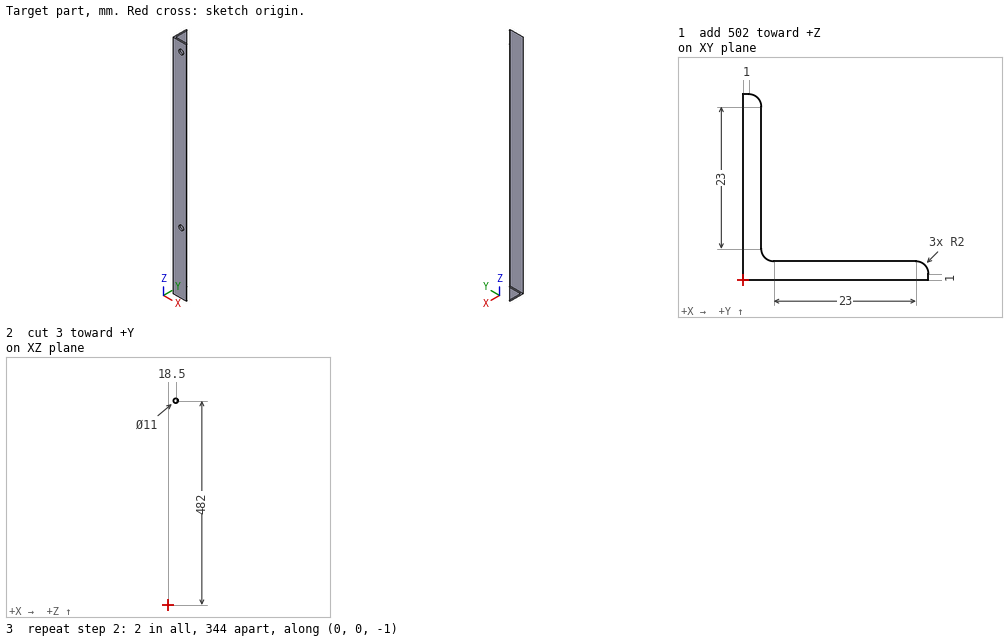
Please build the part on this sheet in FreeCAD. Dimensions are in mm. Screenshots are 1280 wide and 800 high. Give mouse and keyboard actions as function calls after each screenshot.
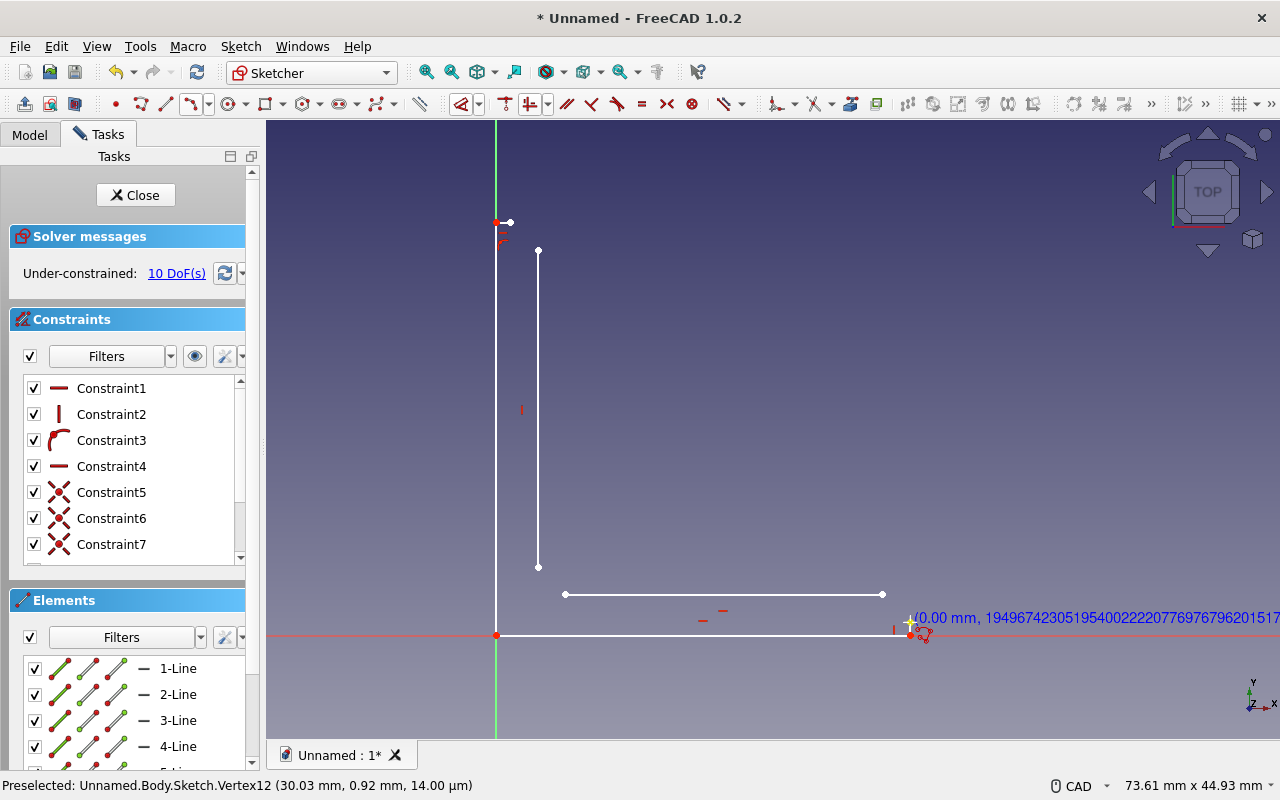
key(g)
key(3)
key(a)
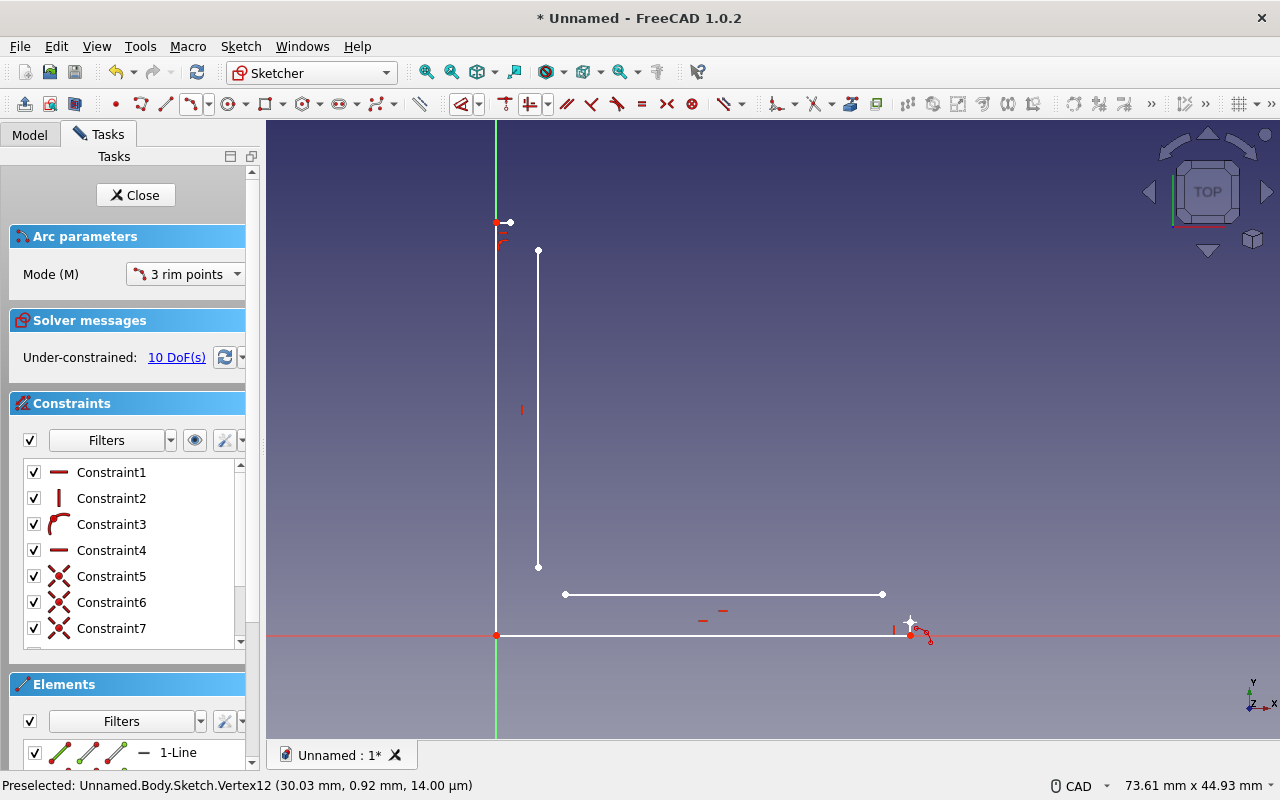
click(565, 595)
click(538, 568)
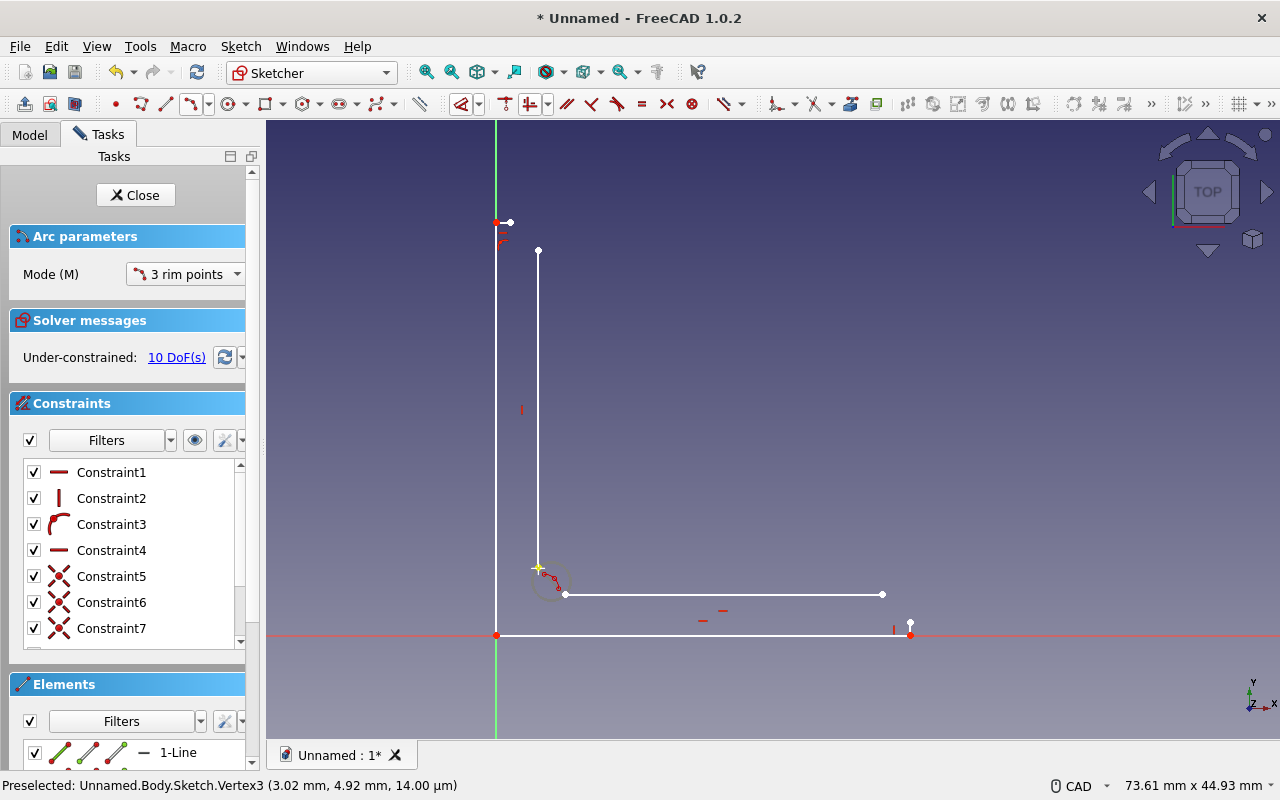
scroll(546, 586, up, 4)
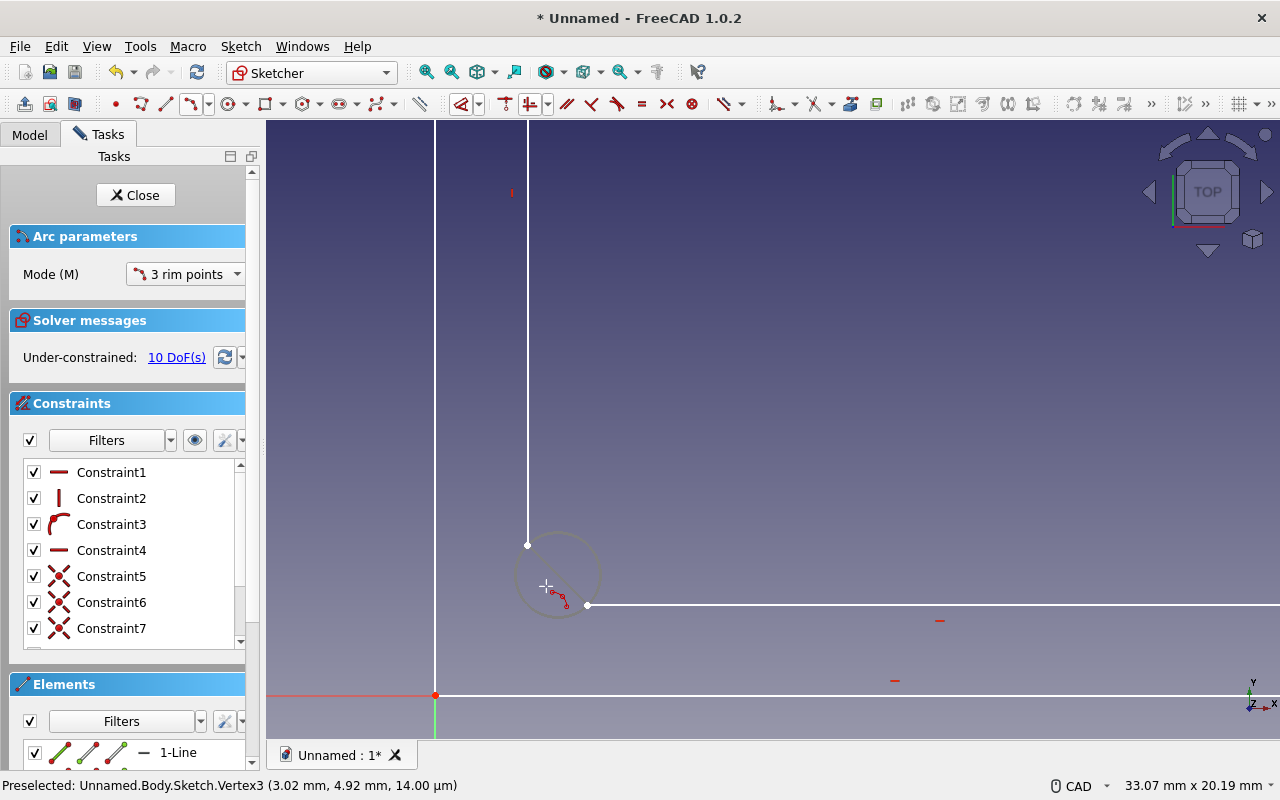
click(545, 586)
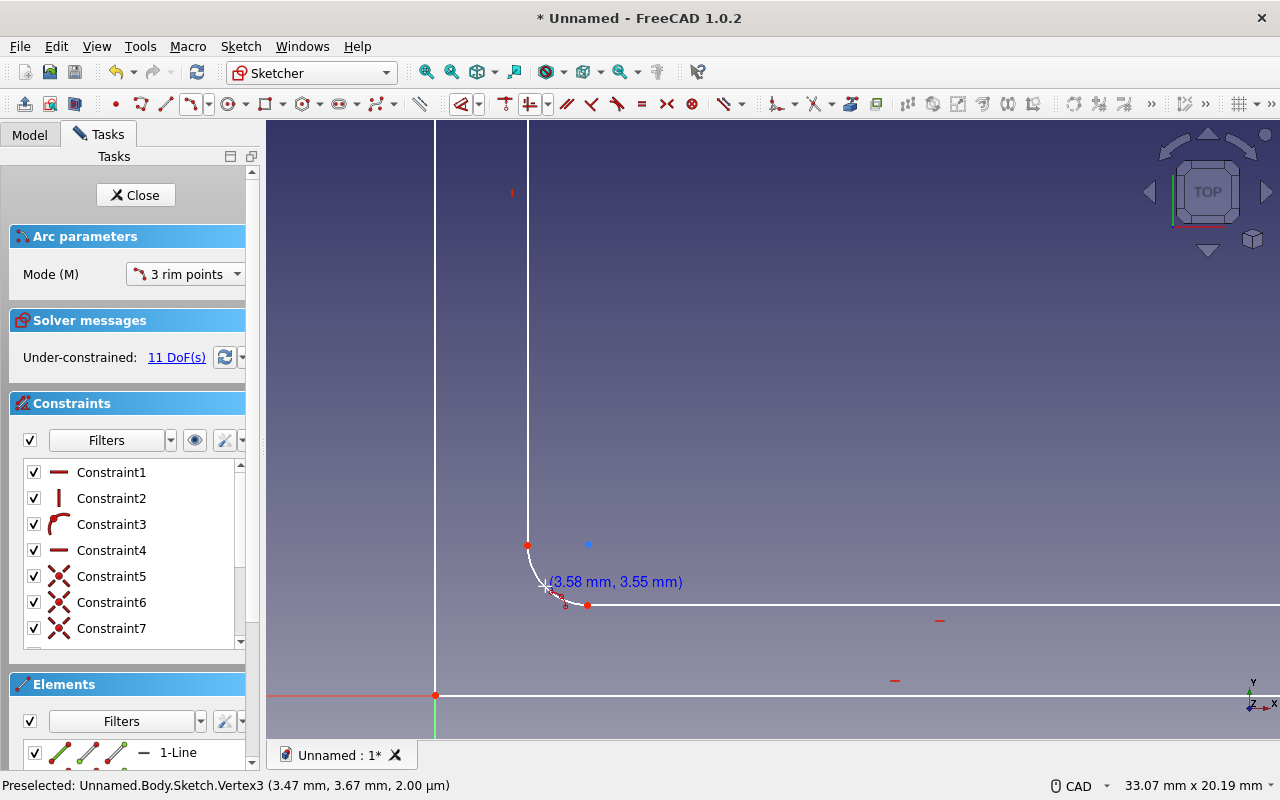
scroll(549, 588, down, 4)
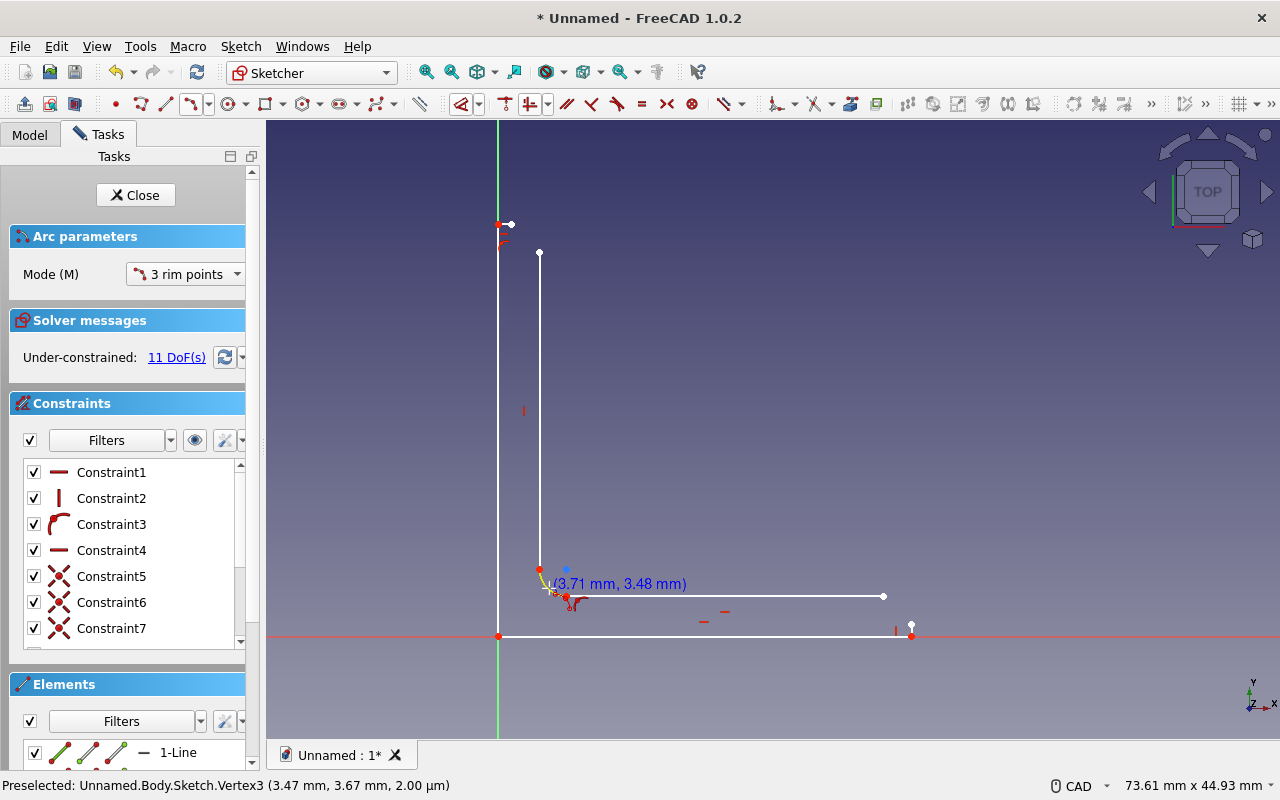
click(540, 252)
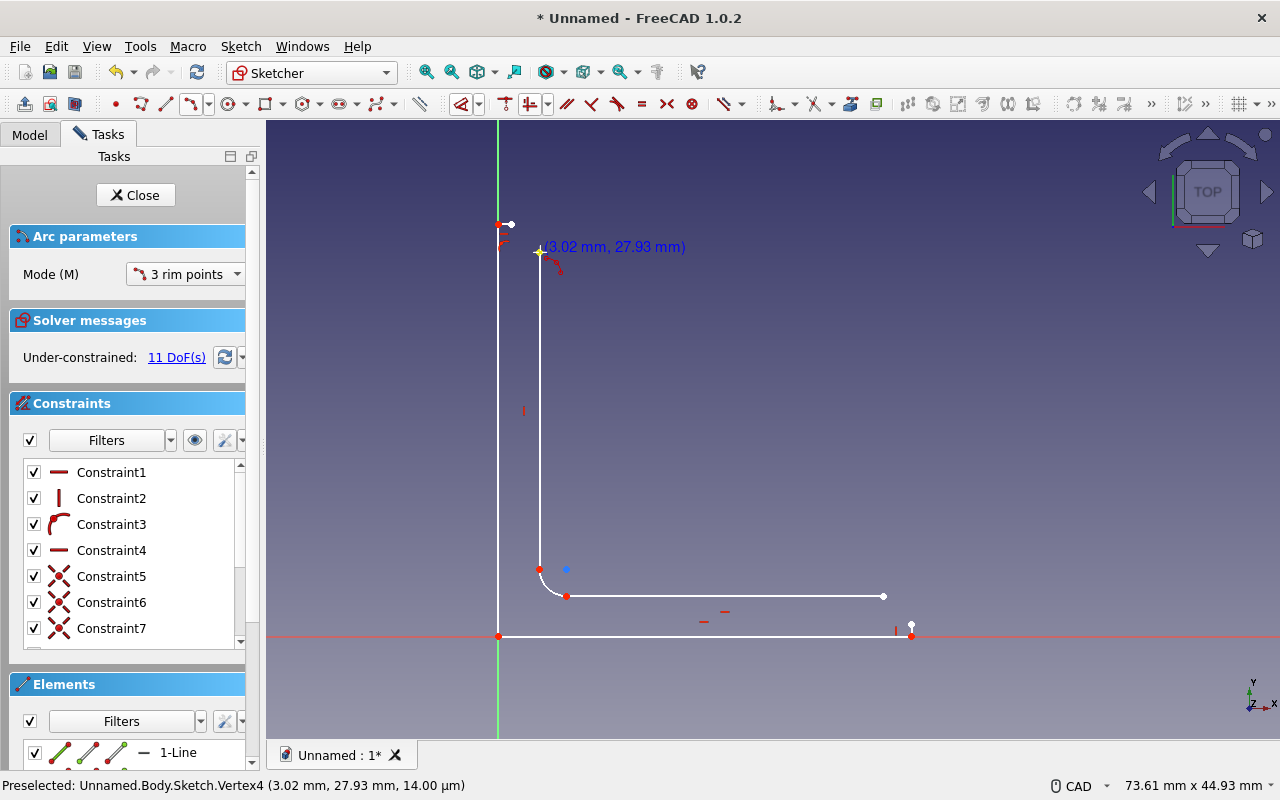
scroll(512, 224, up, 5)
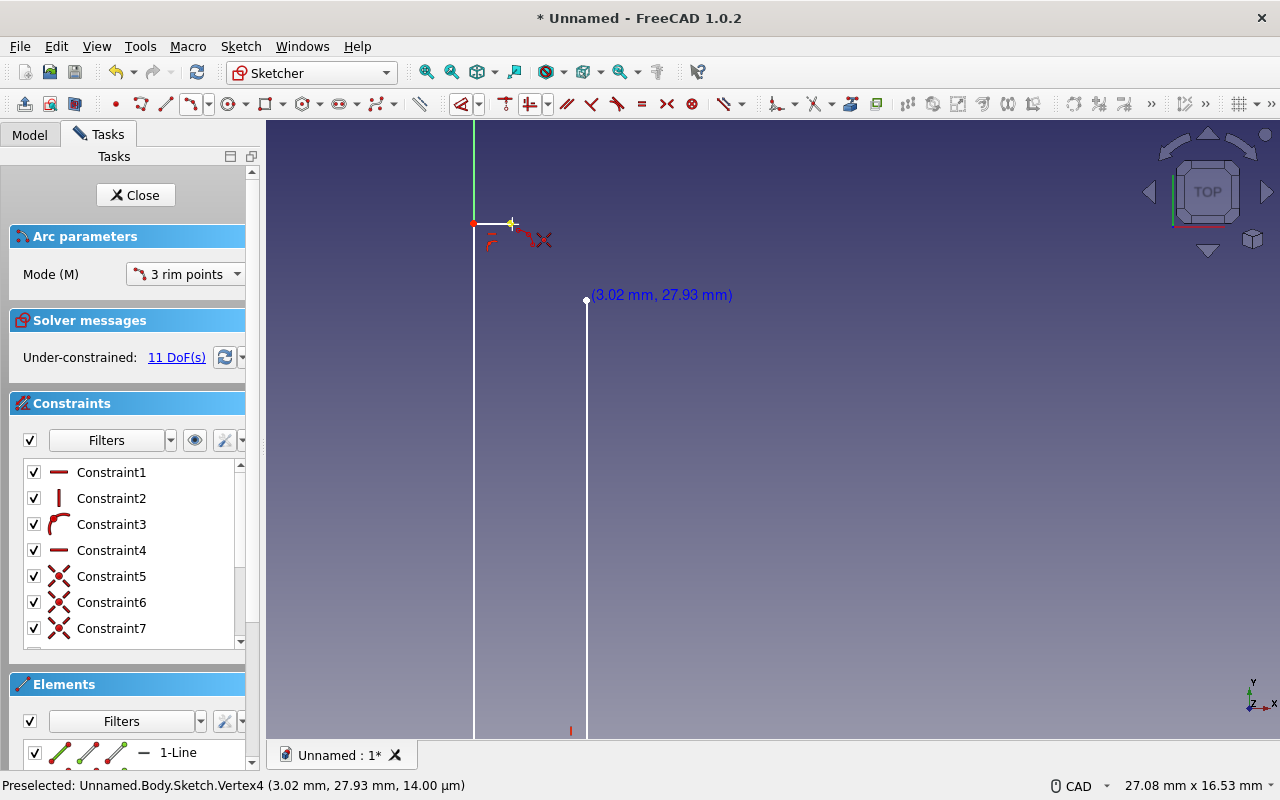
click(511, 224)
click(564, 244)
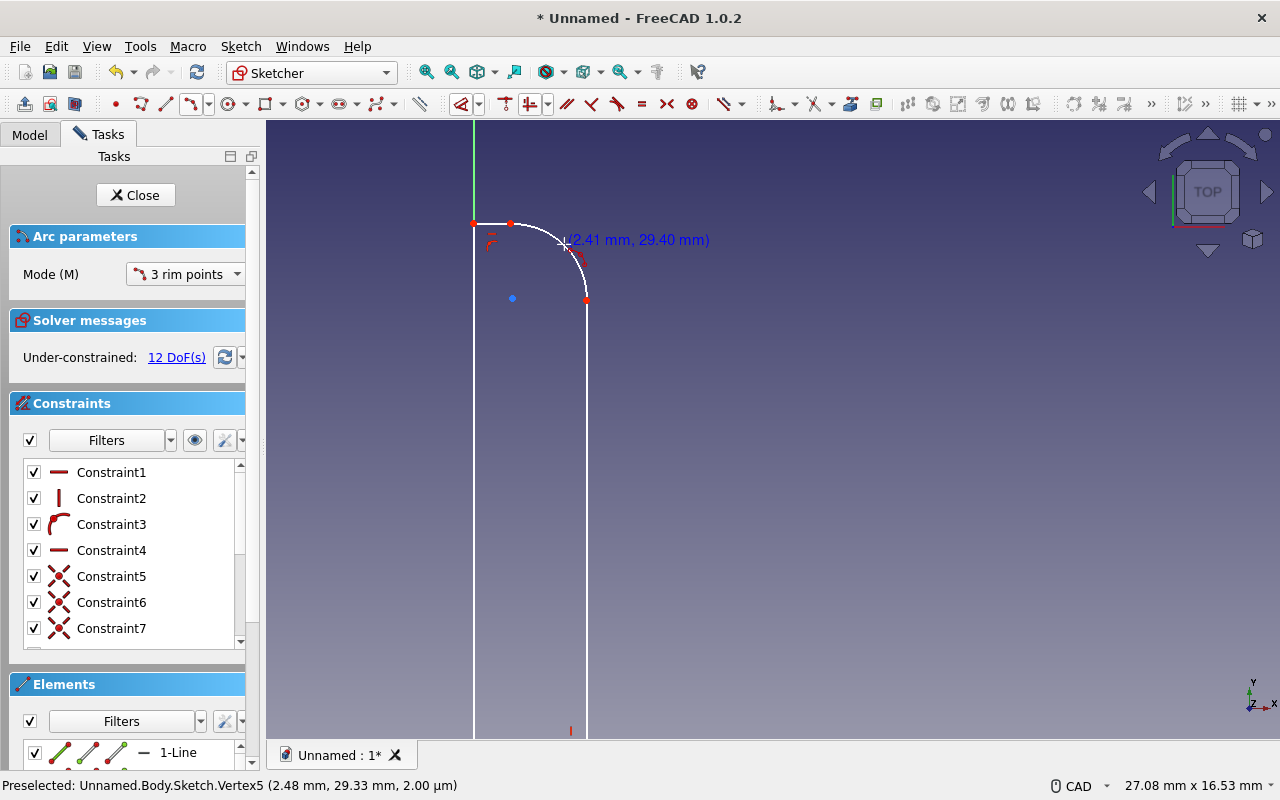
scroll(512, 223, down, 5)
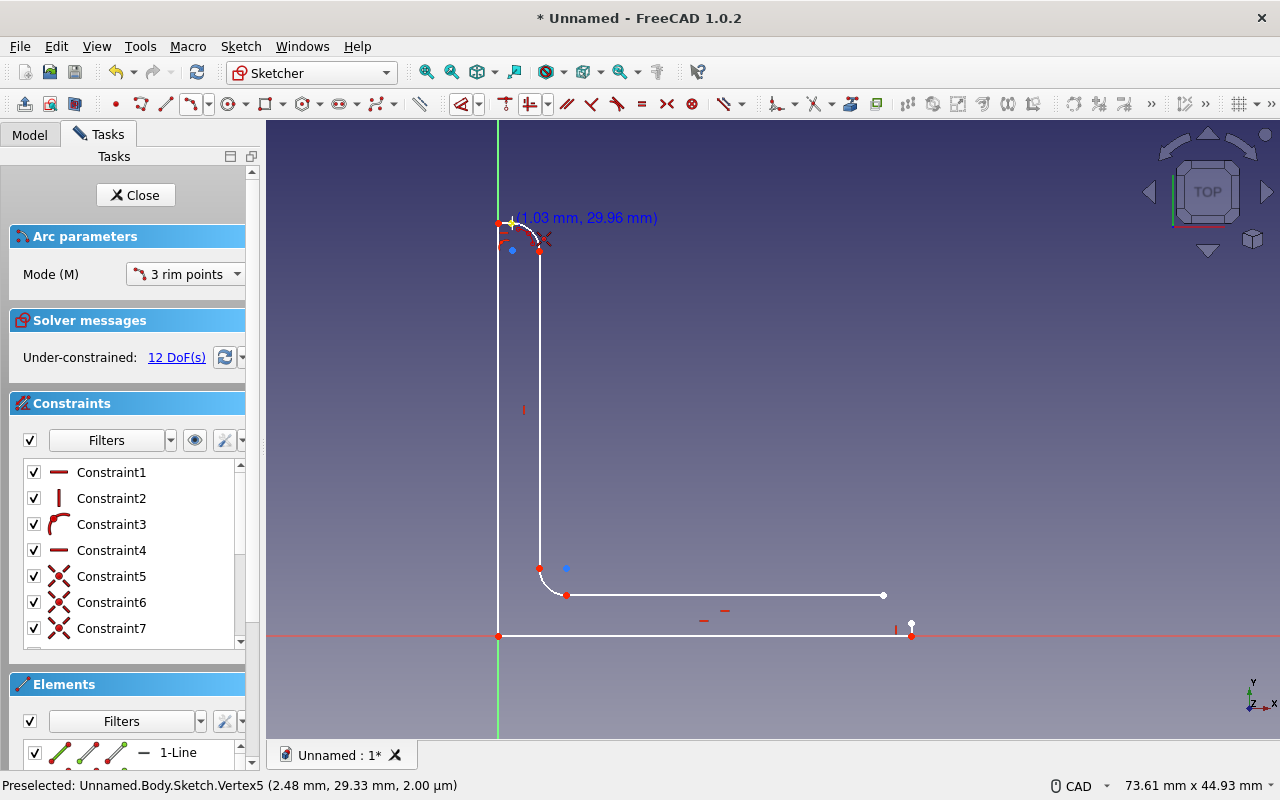
scroll(911, 622, up, 5)